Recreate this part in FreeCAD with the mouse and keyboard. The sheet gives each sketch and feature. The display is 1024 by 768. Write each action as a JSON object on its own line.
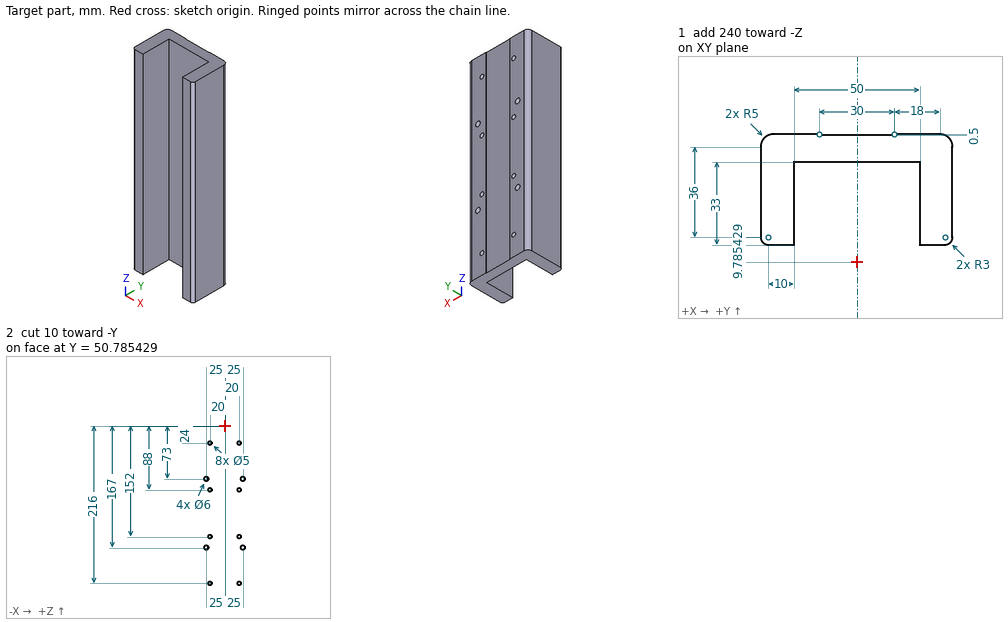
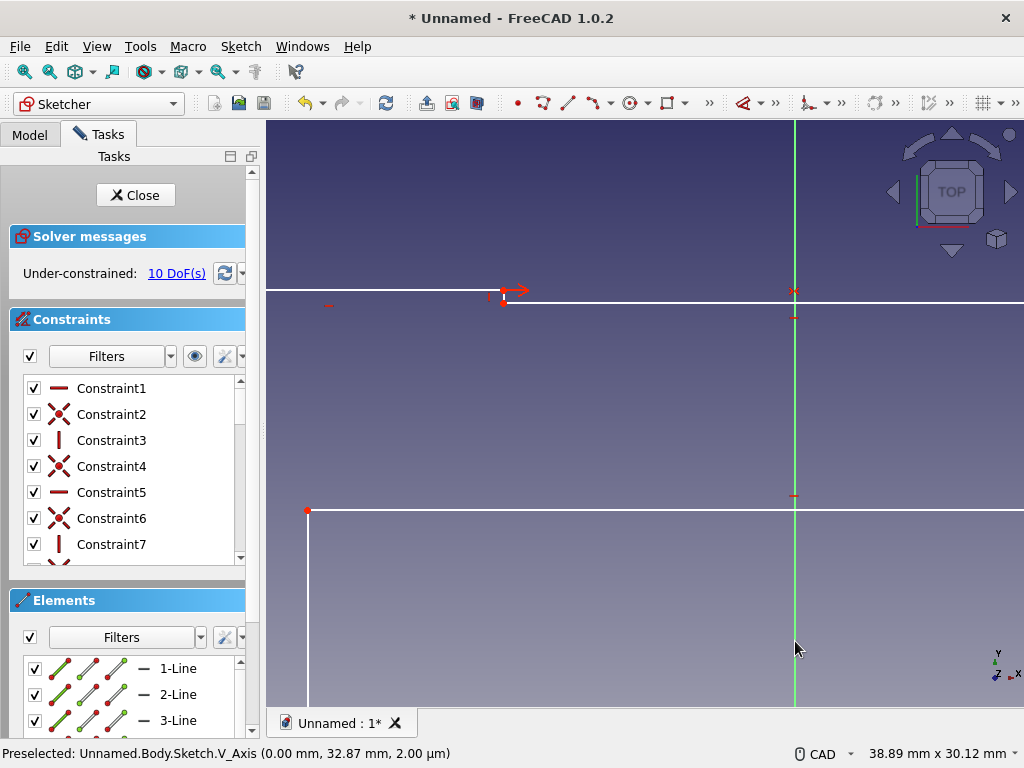
{"action": "scroll", "coordinate": [505, 291], "scroll_direction": "down", "scroll_amount": 7}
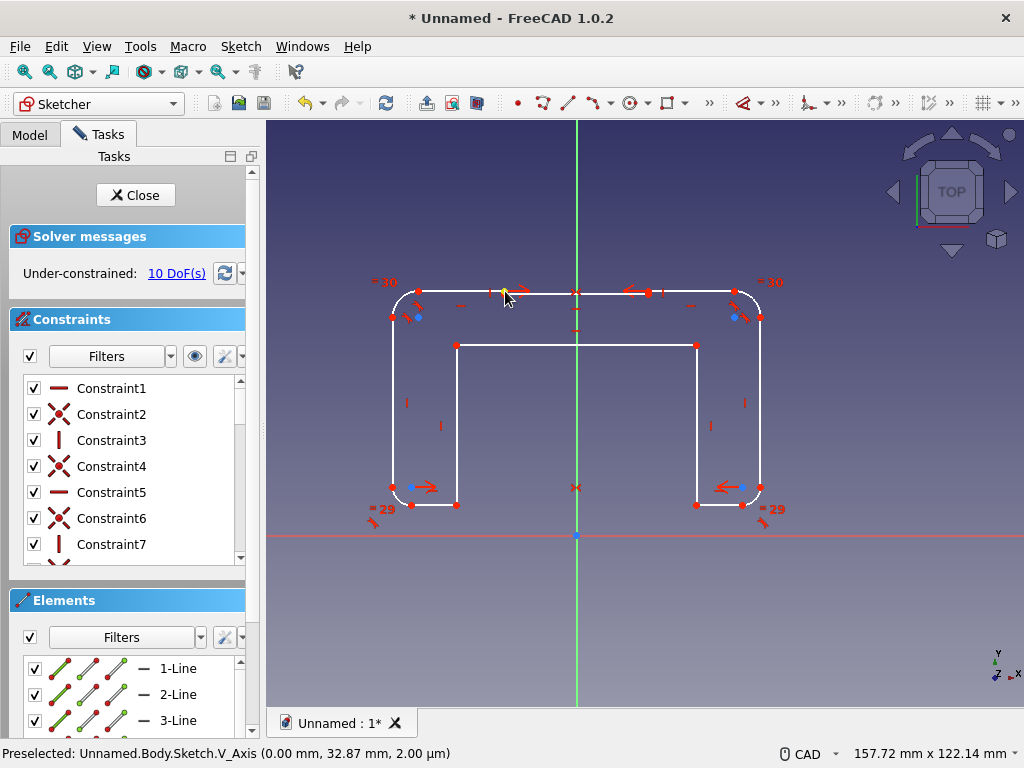
{"action": "scroll", "coordinate": [407, 294], "scroll_direction": "up", "scroll_amount": 3}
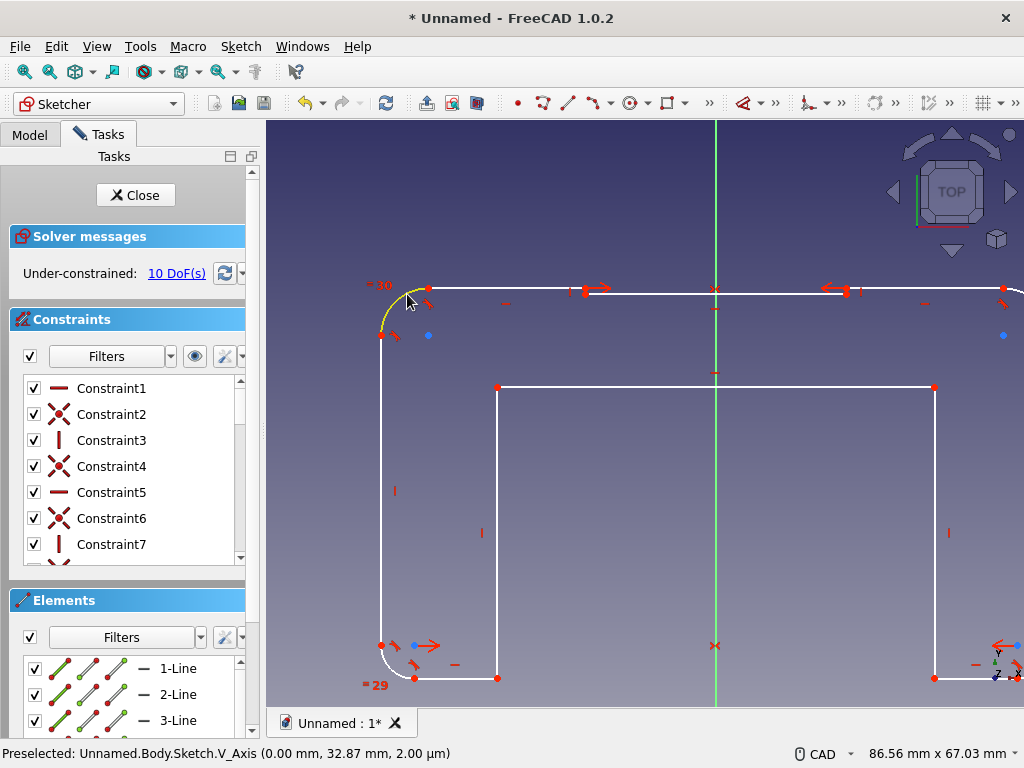
{"action": "left_click", "coordinate": [407, 294]}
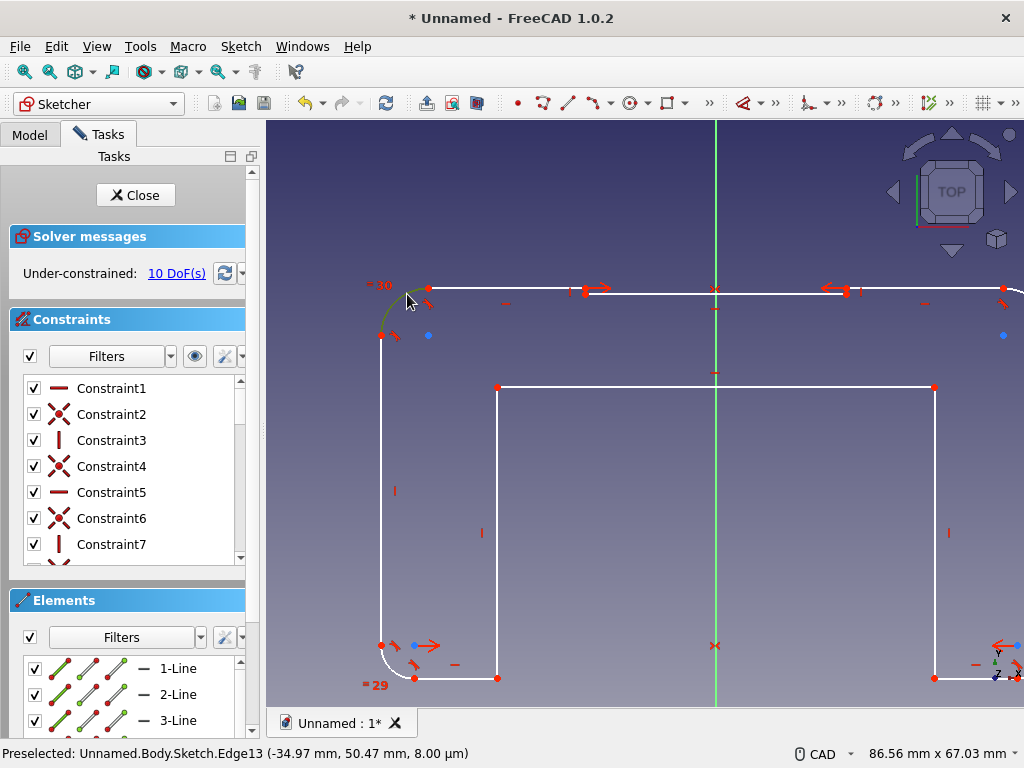
{"action": "key", "text": "k r"}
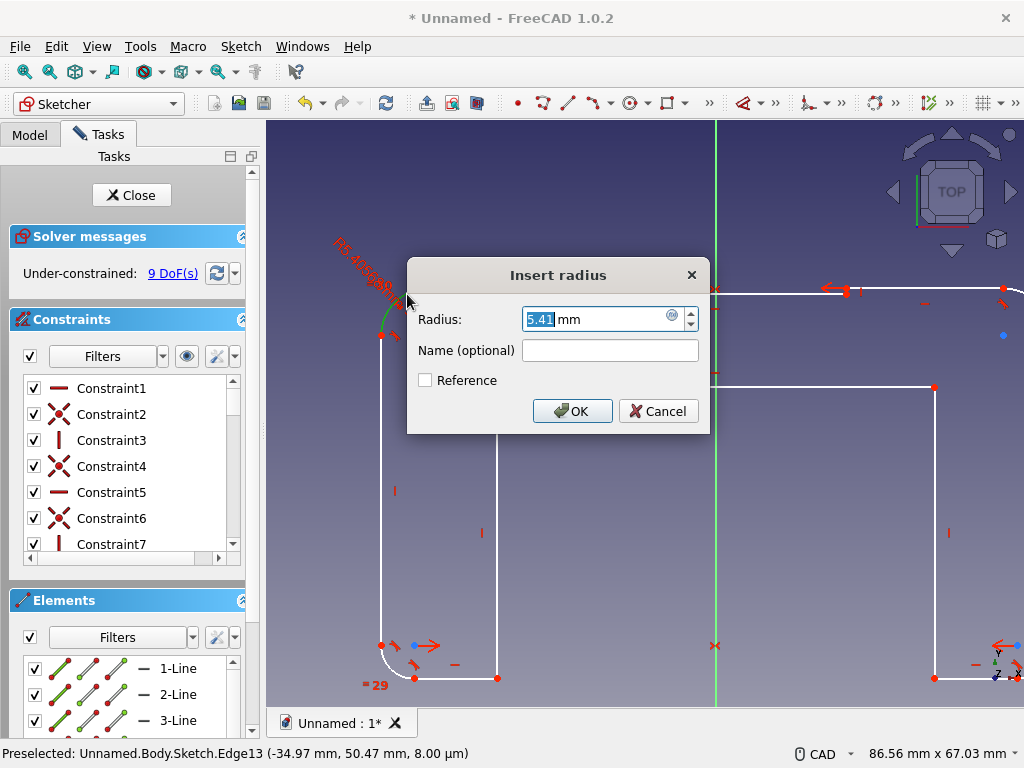
{"action": "type", "text": "5"}
{"action": "key", "text": "Return"}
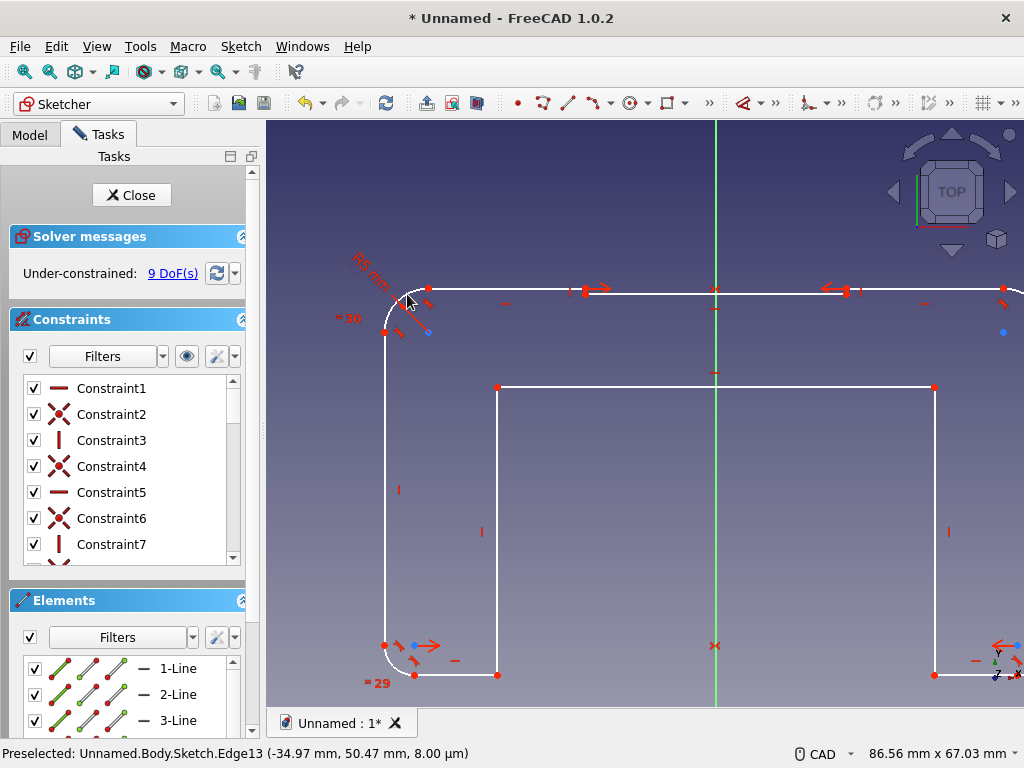
{"action": "scroll", "coordinate": [388, 659], "scroll_direction": "up", "scroll_amount": 3}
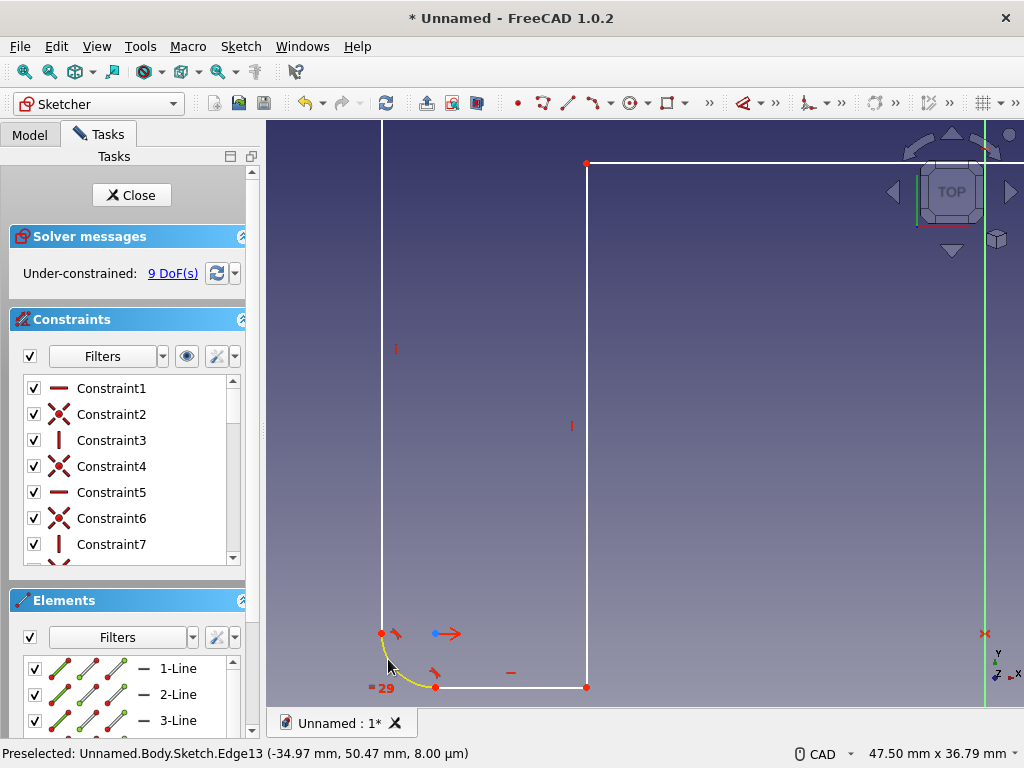
{"action": "left_click", "coordinate": [388, 658]}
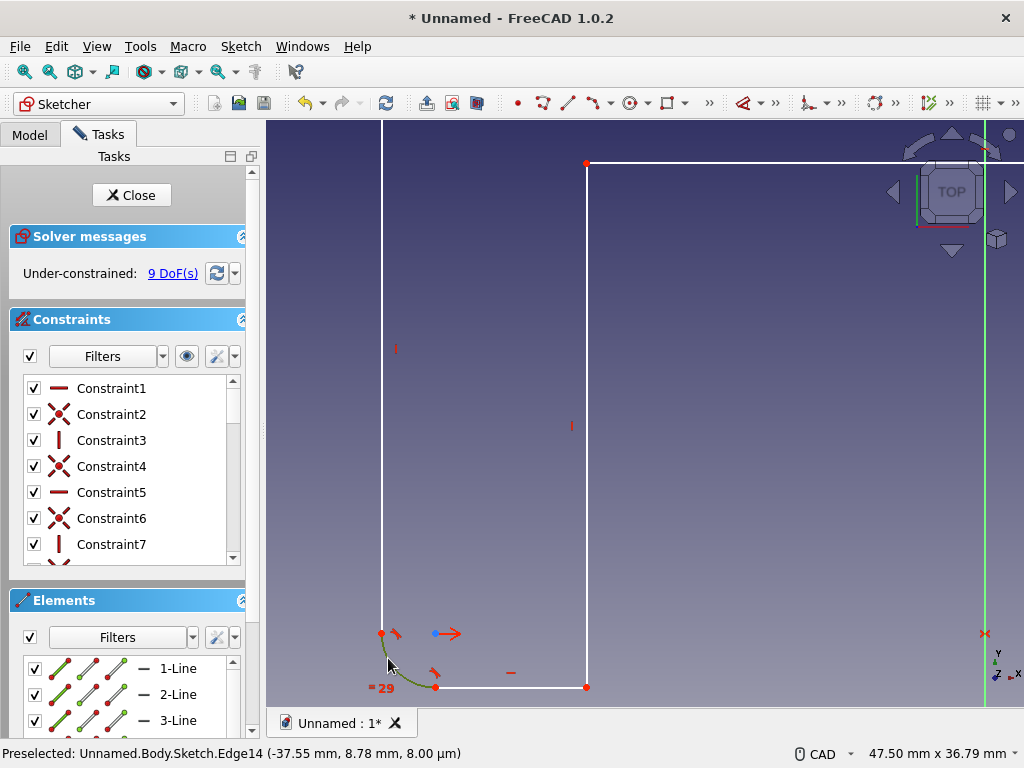
{"action": "key", "text": "k r"}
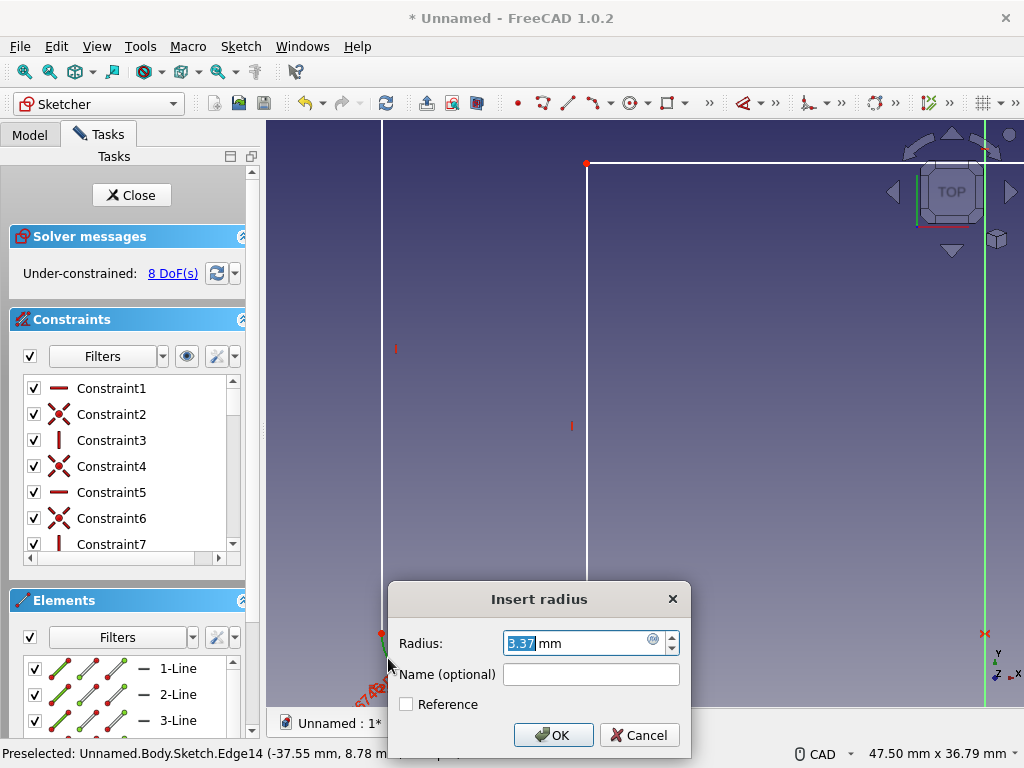
{"action": "type", "text": "3"}
{"action": "key", "text": "Return"}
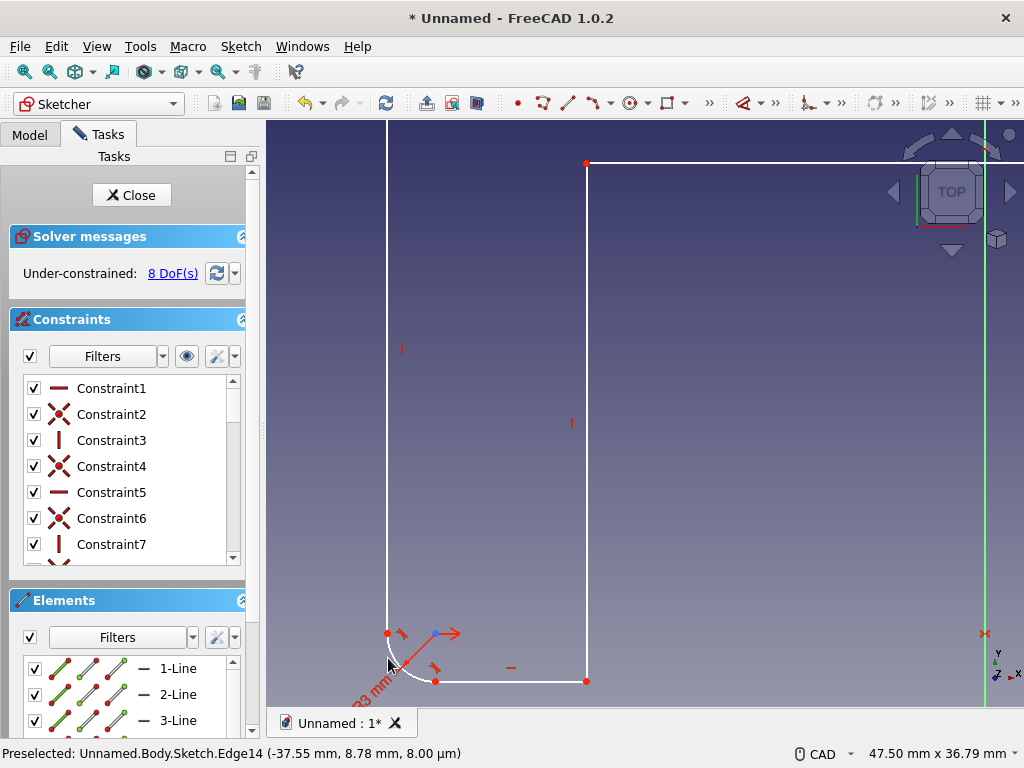
{"action": "scroll", "coordinate": [400, 424], "scroll_direction": "down", "scroll_amount": 6}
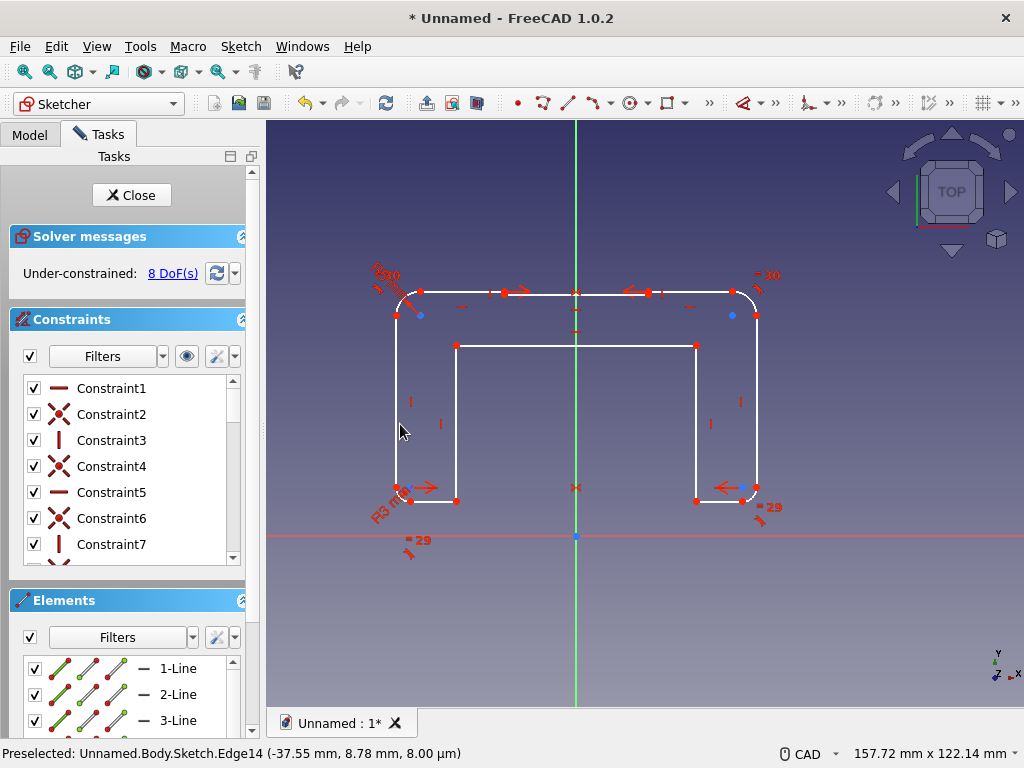
{"action": "left_click", "coordinate": [707, 292]}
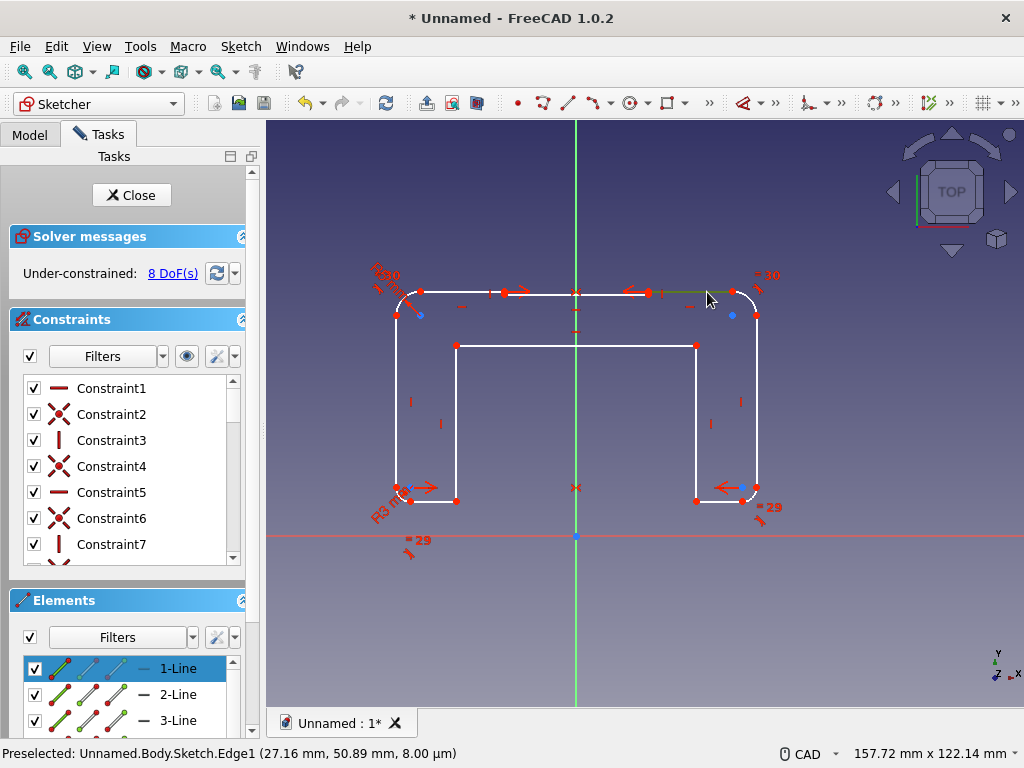
{"action": "key", "text": "l"}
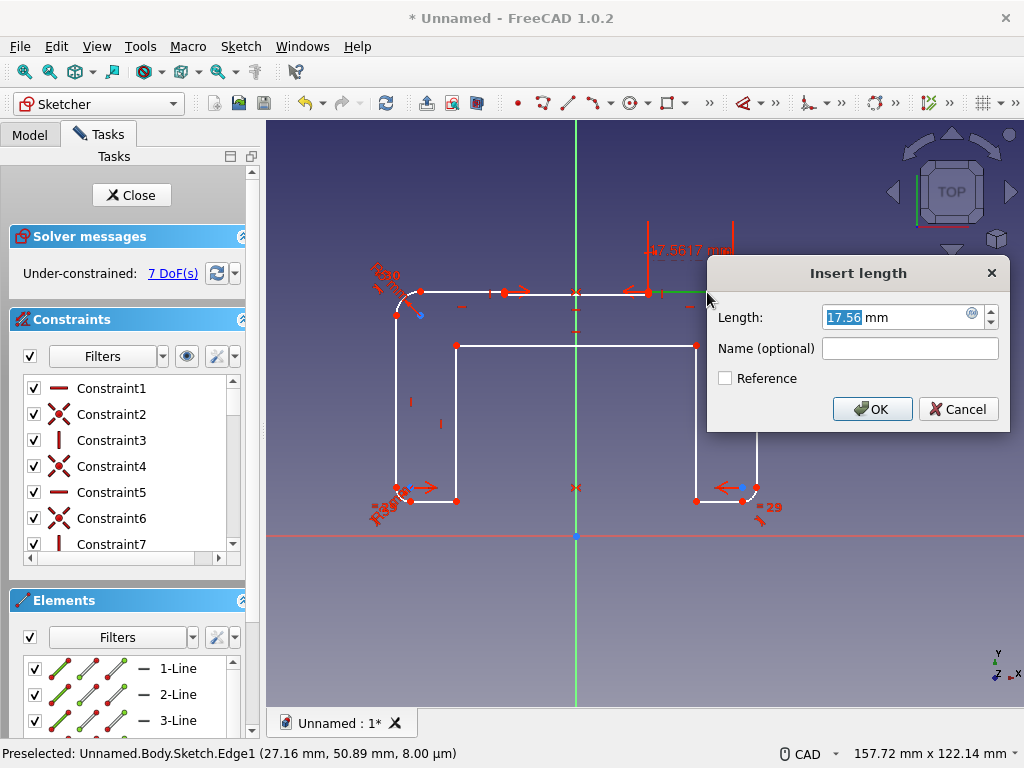
{"action": "type", "text": "18"}
{"action": "key", "text": "Return"}